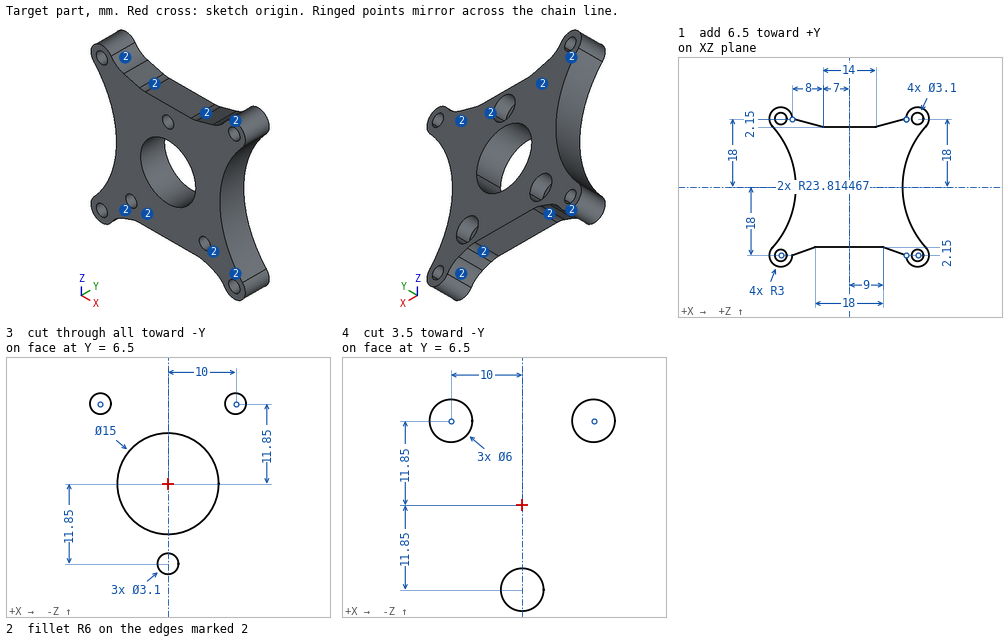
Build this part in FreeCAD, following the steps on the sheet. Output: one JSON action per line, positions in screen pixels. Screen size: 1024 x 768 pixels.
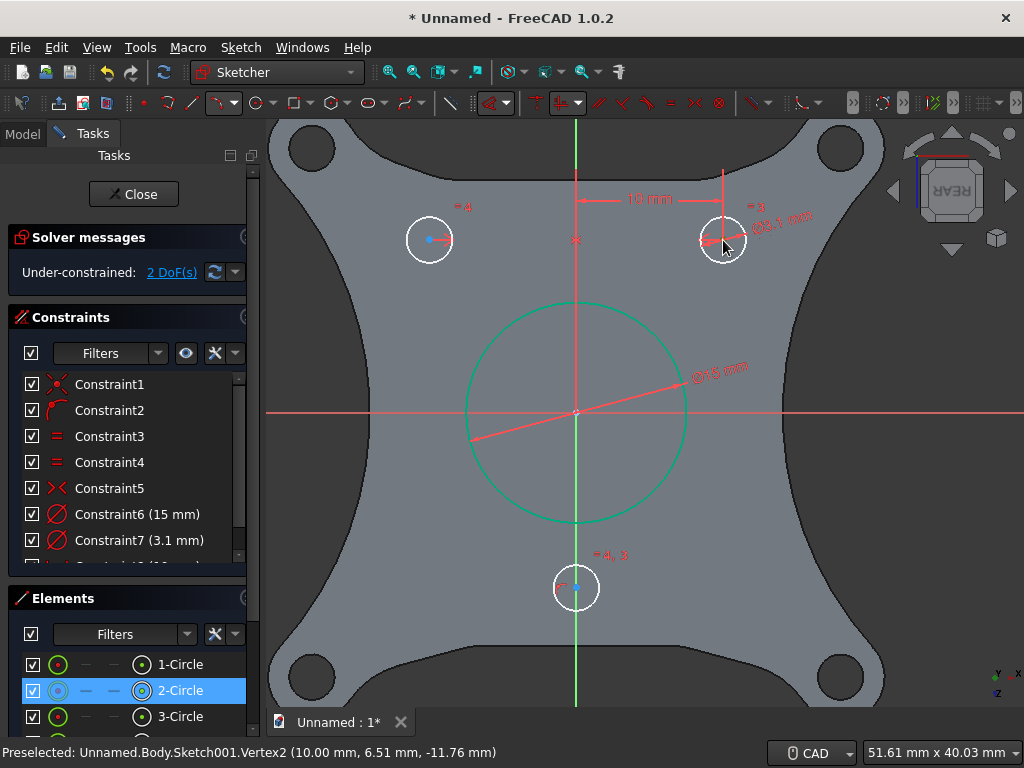
{"action": "key", "text": "i"}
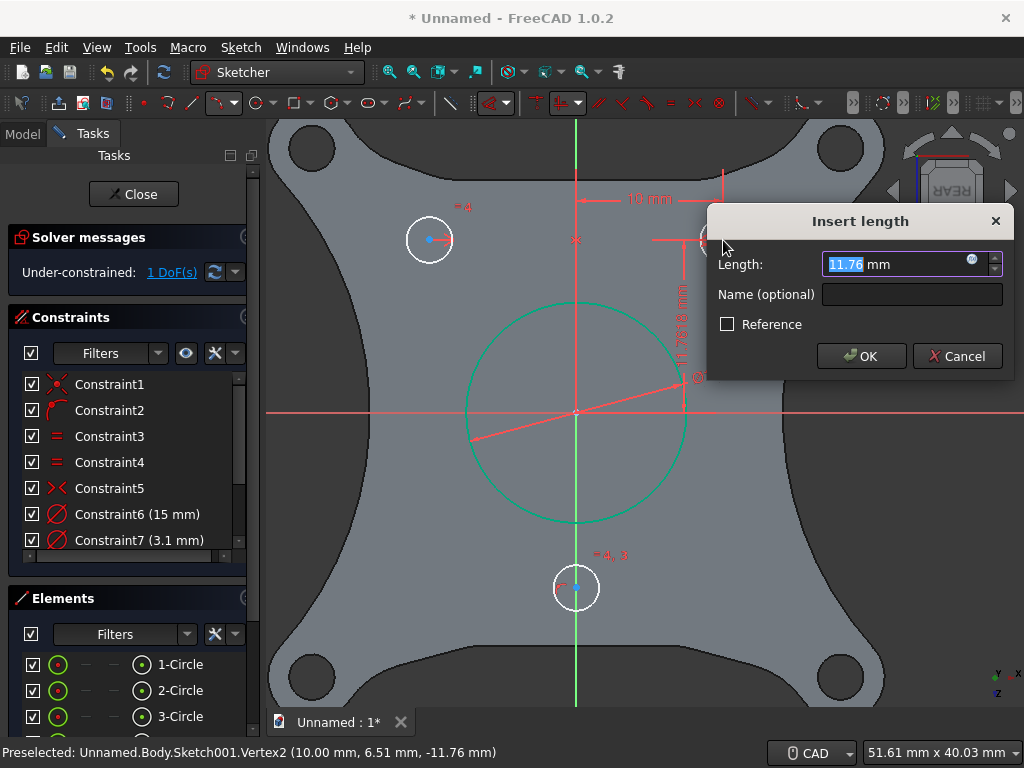
{"action": "type", "text": "11.85"}
{"action": "key", "text": "Return"}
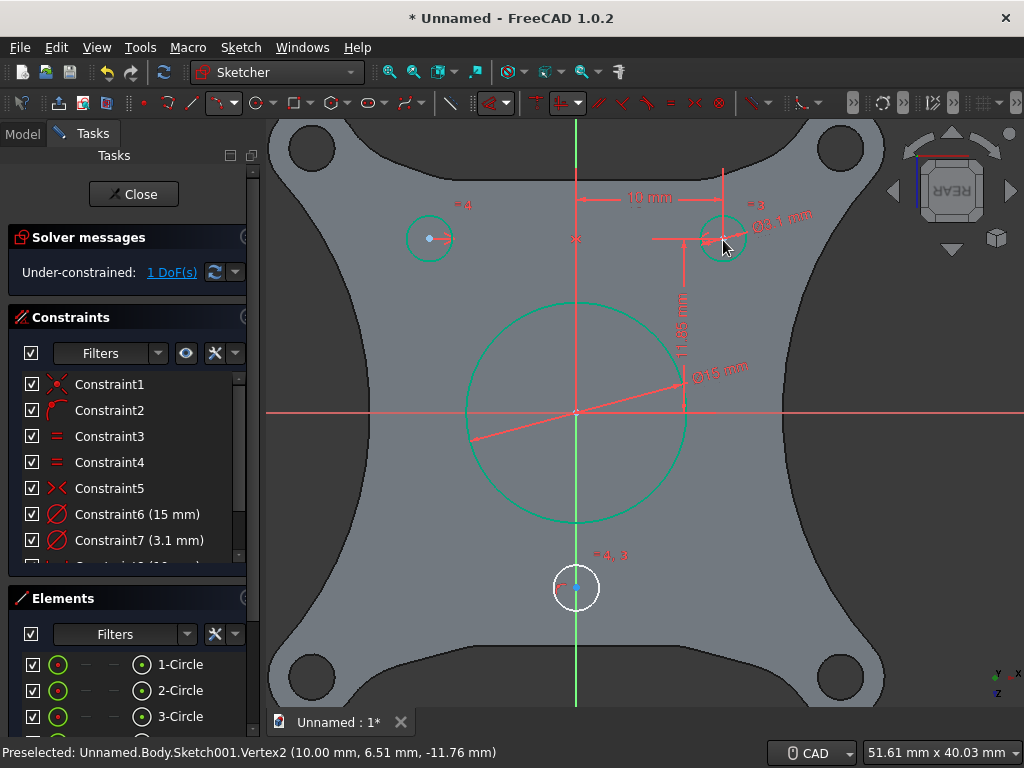
{"action": "left_click", "coordinate": [576, 588]}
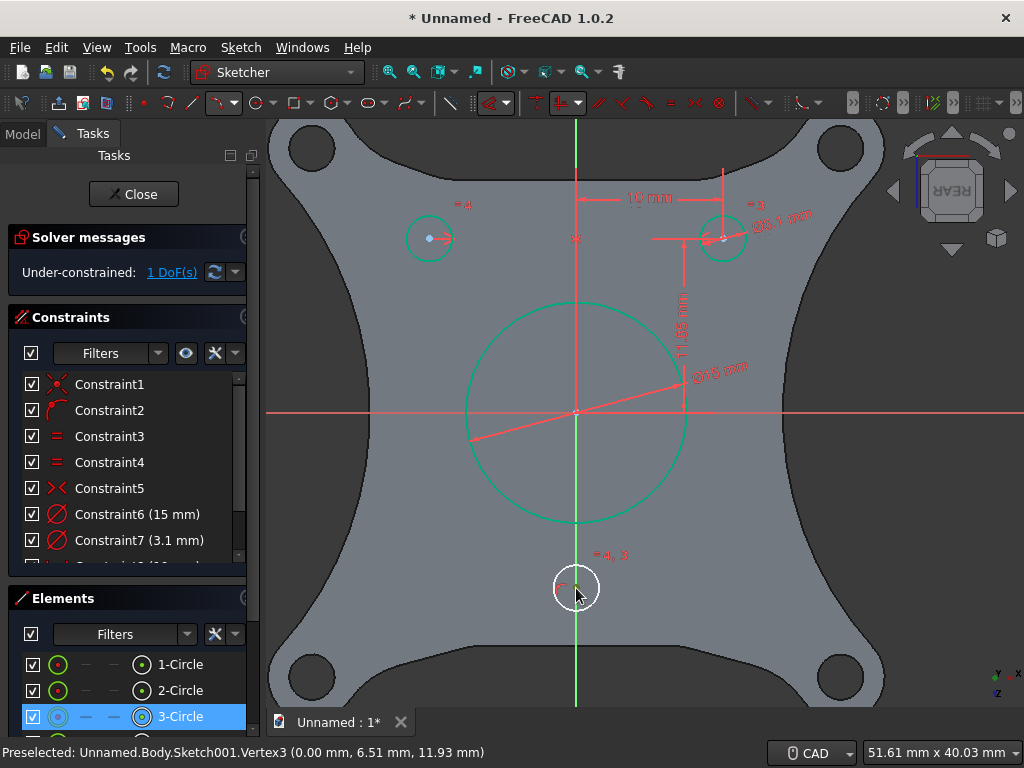
{"action": "key", "text": "i"}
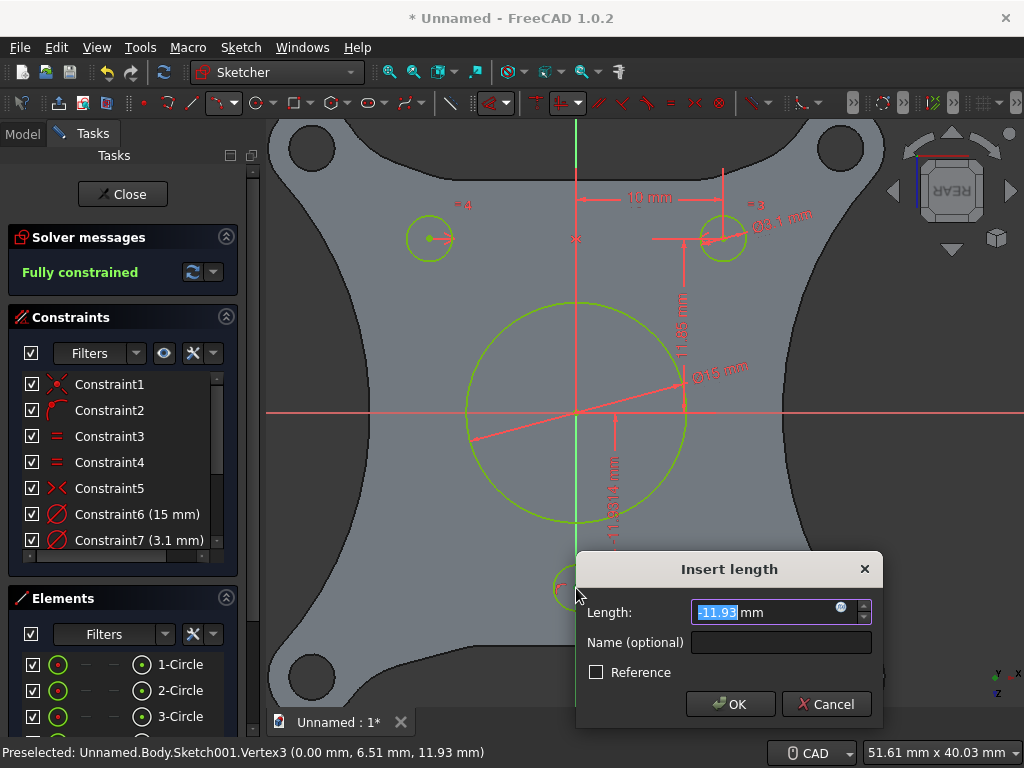
{"action": "type", "text": "-11.85"}
{"action": "key", "text": "Return"}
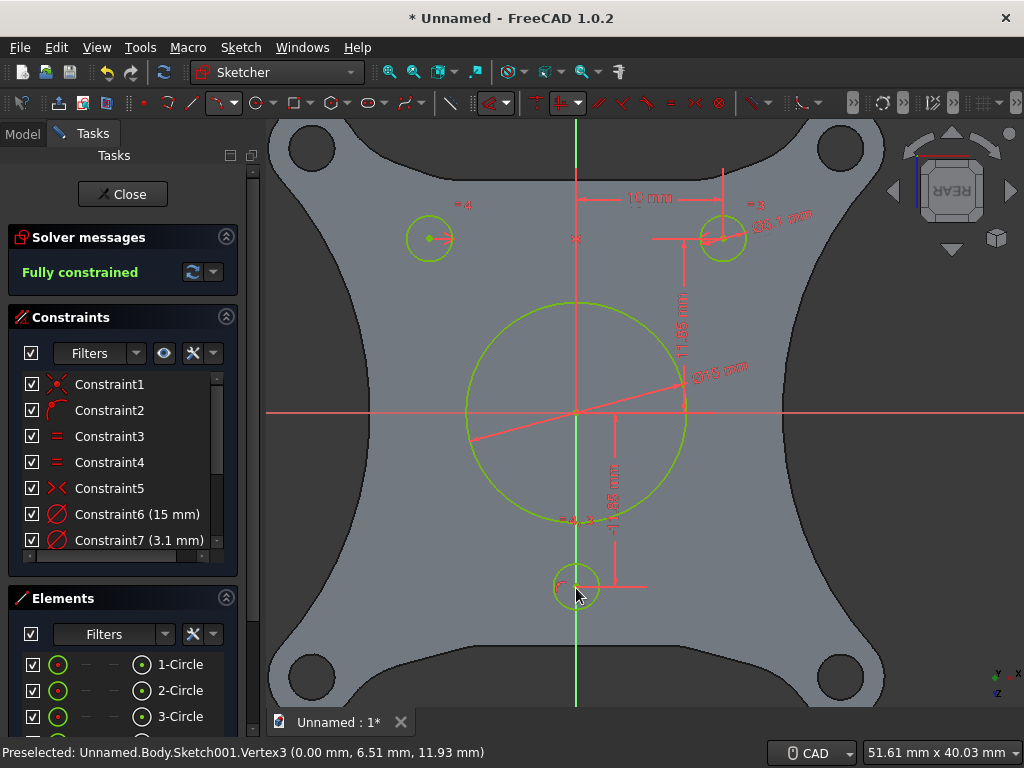
{"action": "left_click", "coordinate": [123, 194]}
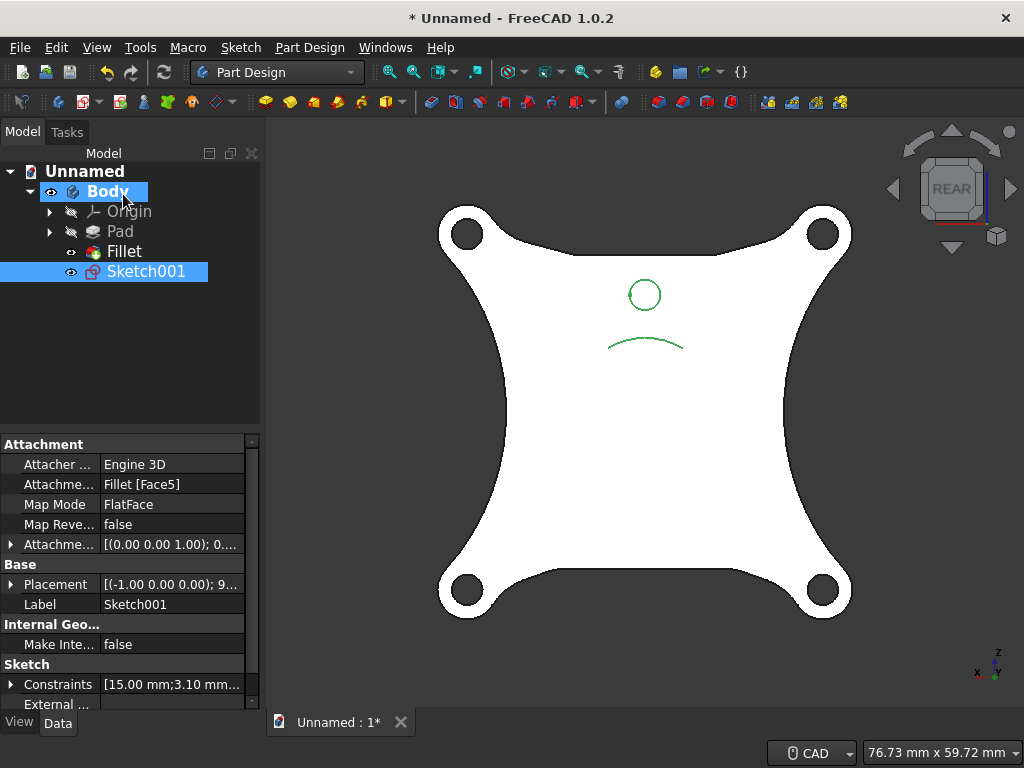
{"action": "left_click", "coordinate": [432, 102]}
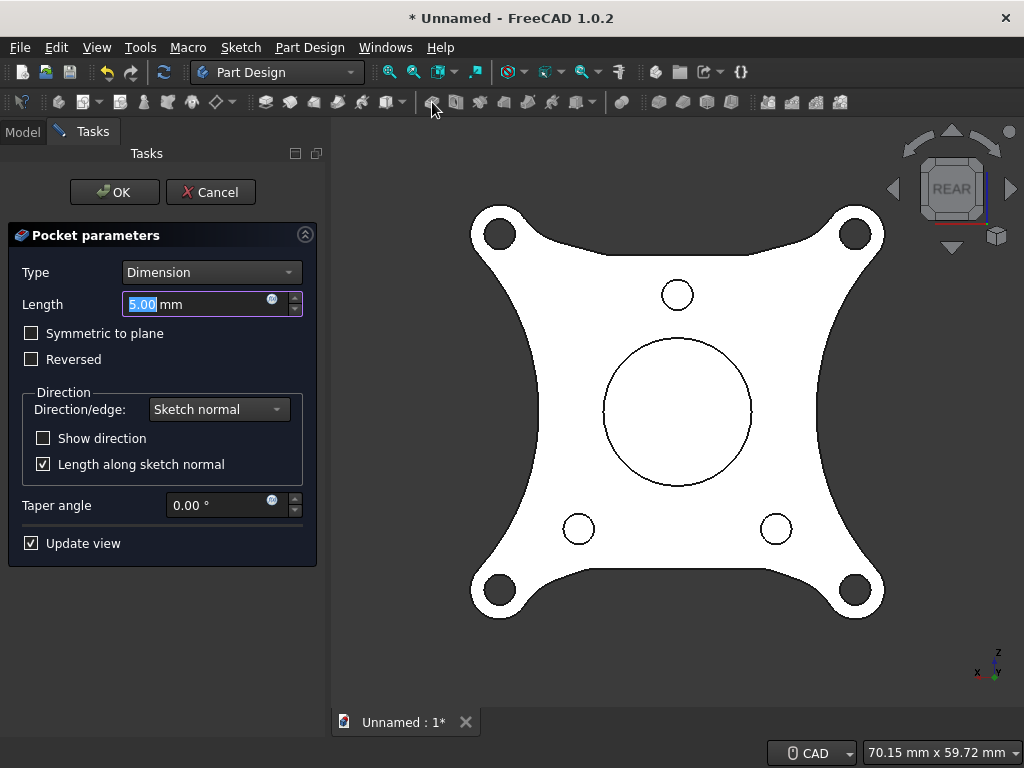
{"action": "left_click", "coordinate": [212, 272]}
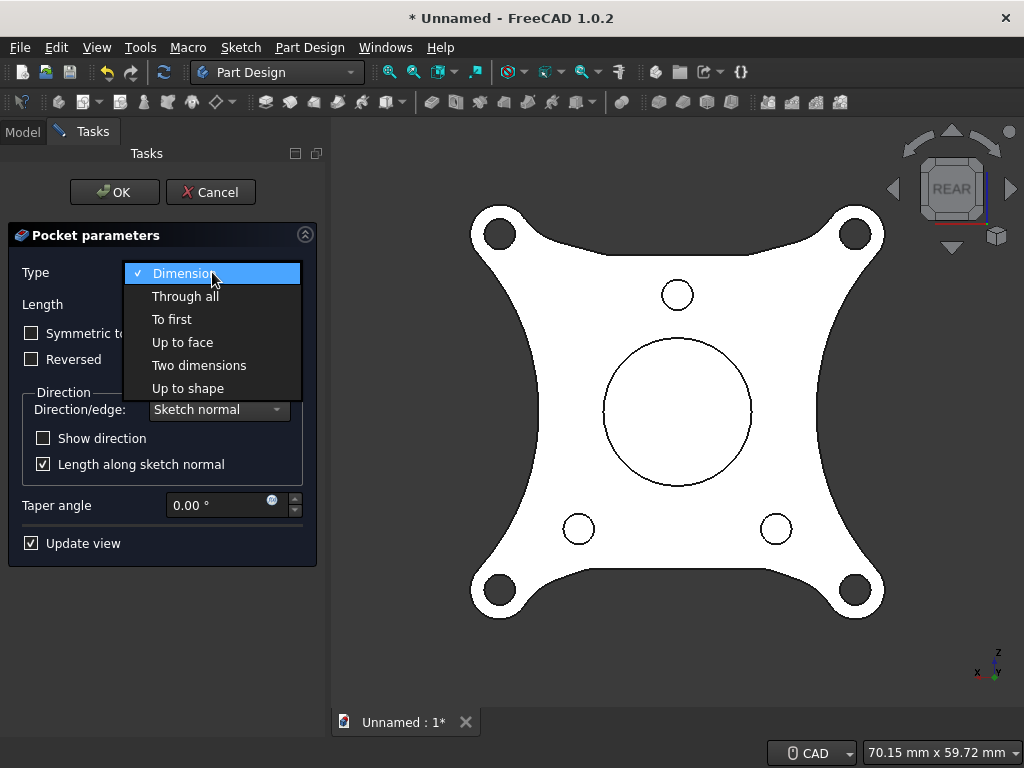
{"action": "left_click", "coordinate": [212, 296]}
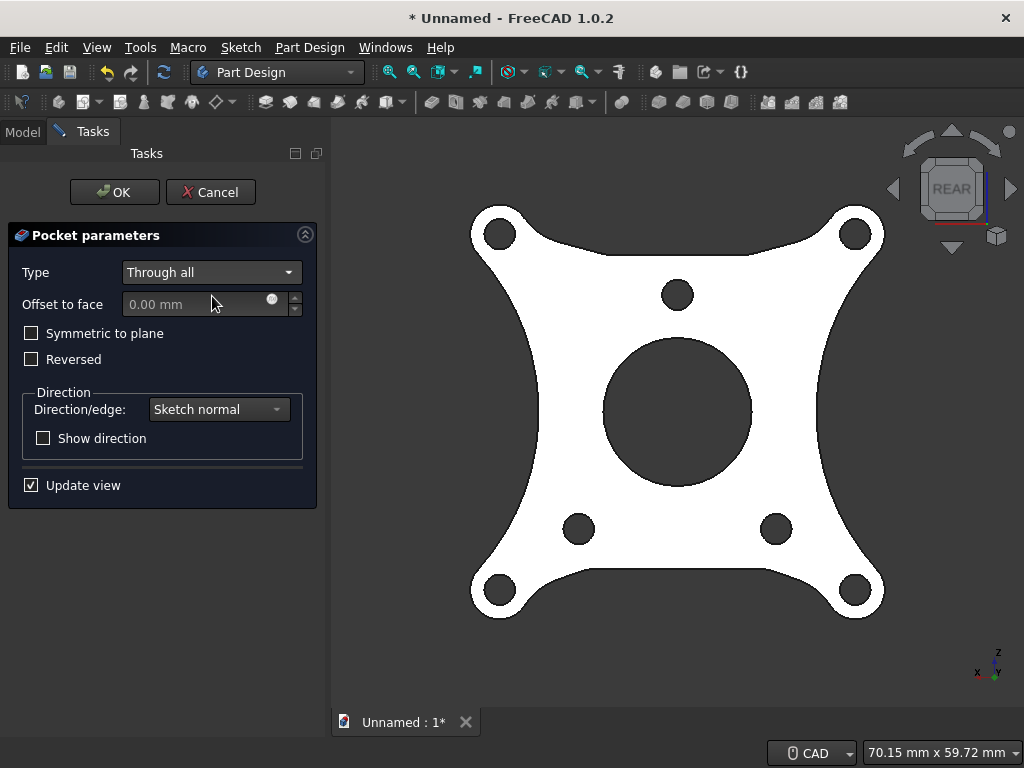
{"action": "left_click", "coordinate": [115, 192]}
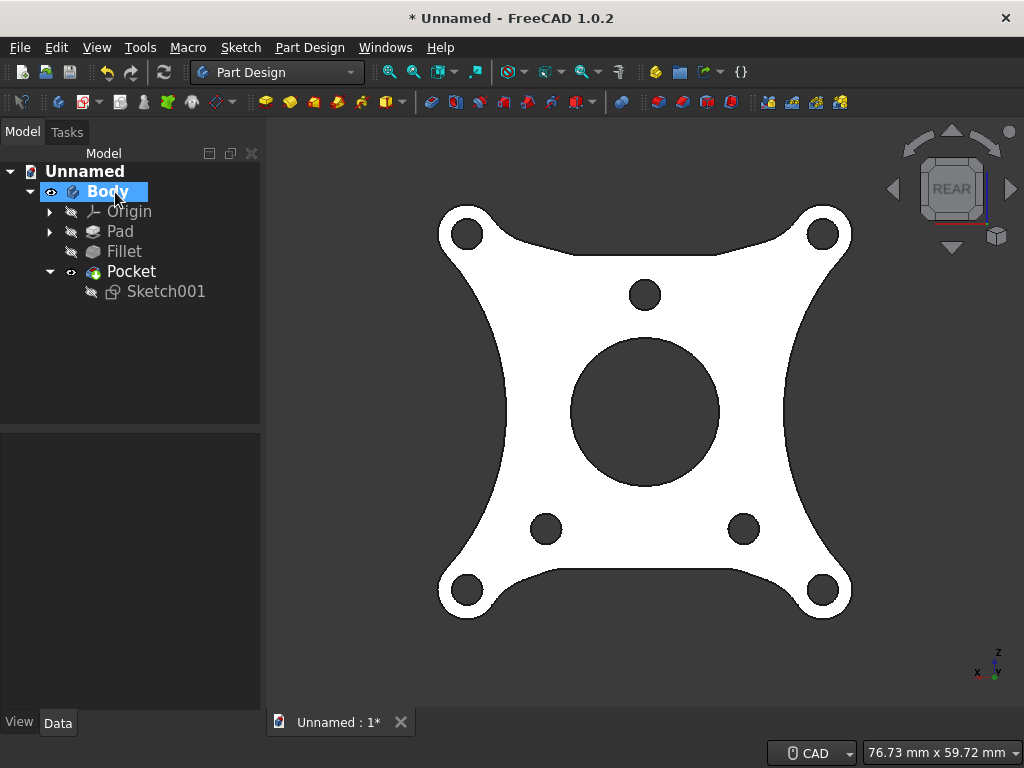
{"action": "left_click", "coordinate": [764, 292]}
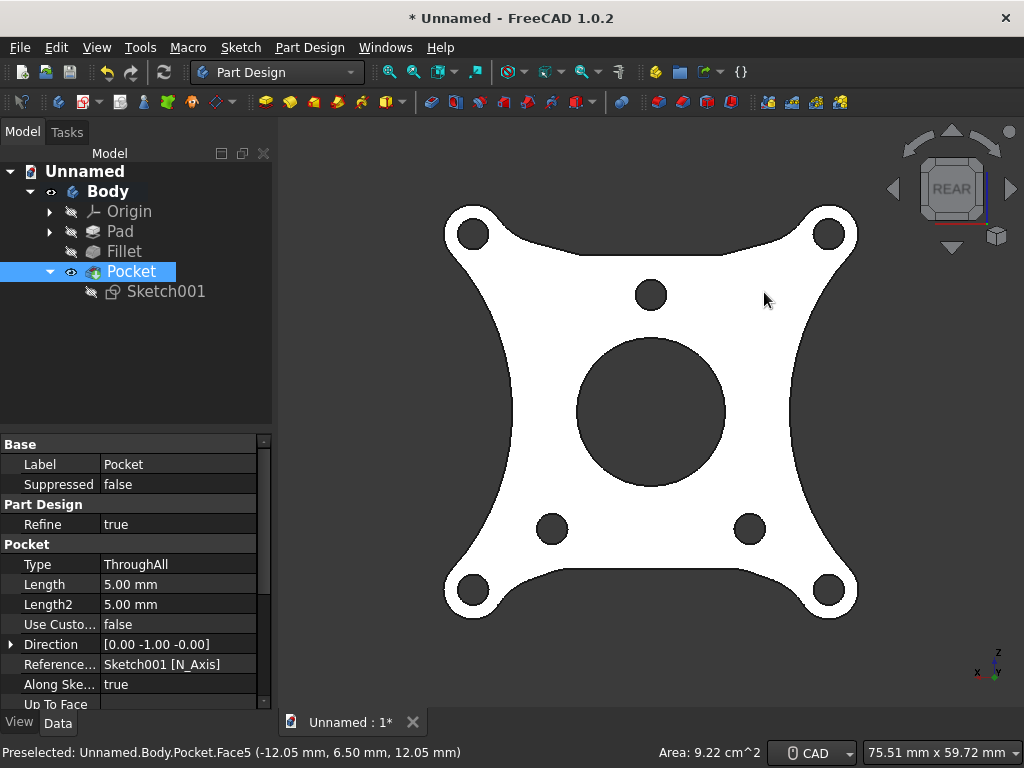
{"action": "left_click", "coordinate": [84, 102]}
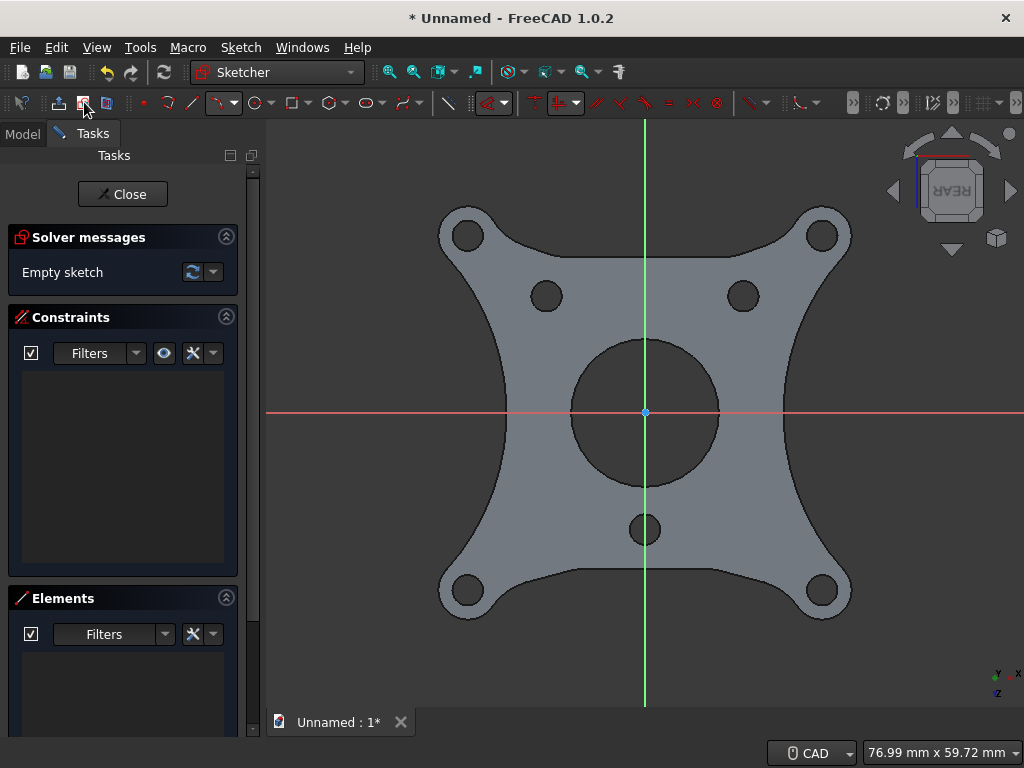
{"action": "left_click", "coordinate": [256, 104]}